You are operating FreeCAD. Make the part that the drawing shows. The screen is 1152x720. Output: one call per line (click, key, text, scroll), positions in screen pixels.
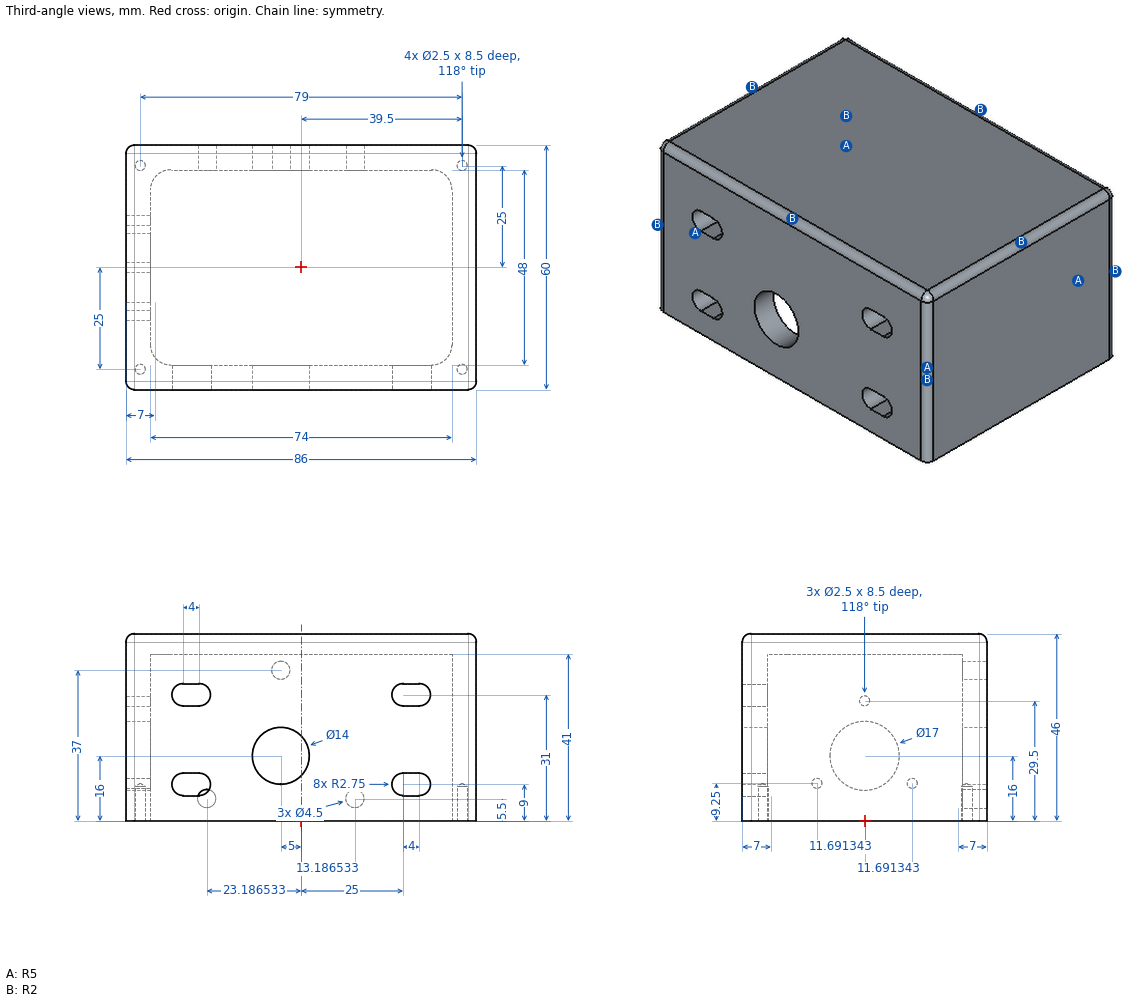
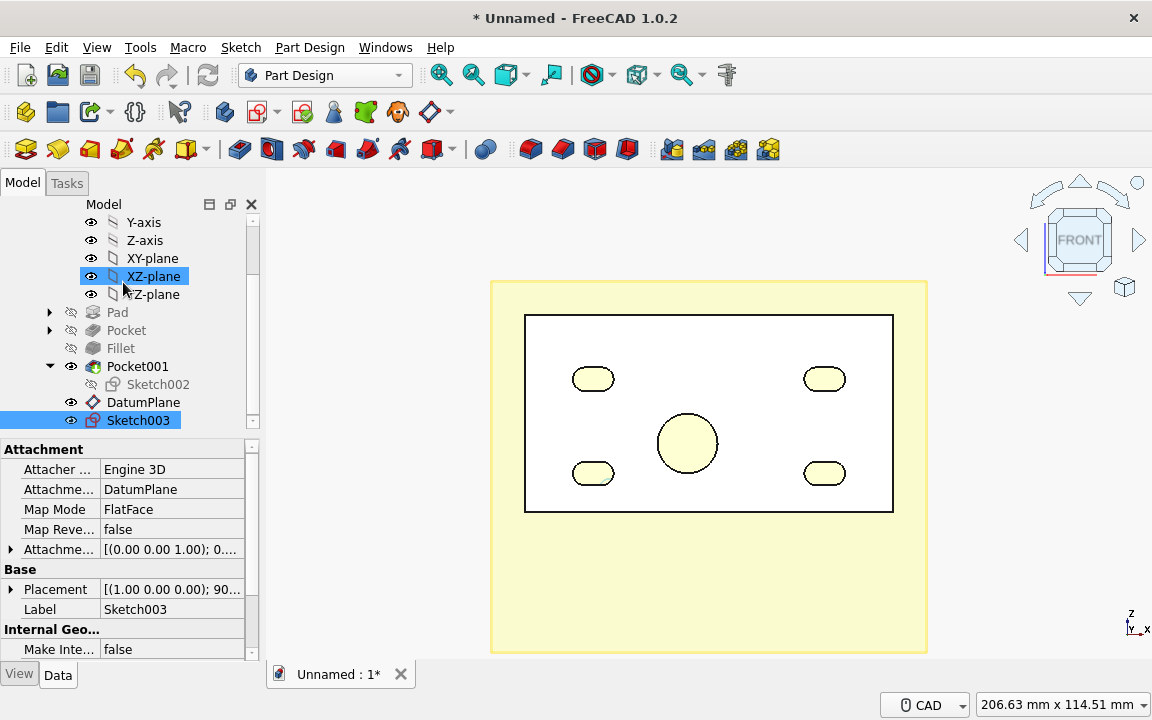
click(240, 150)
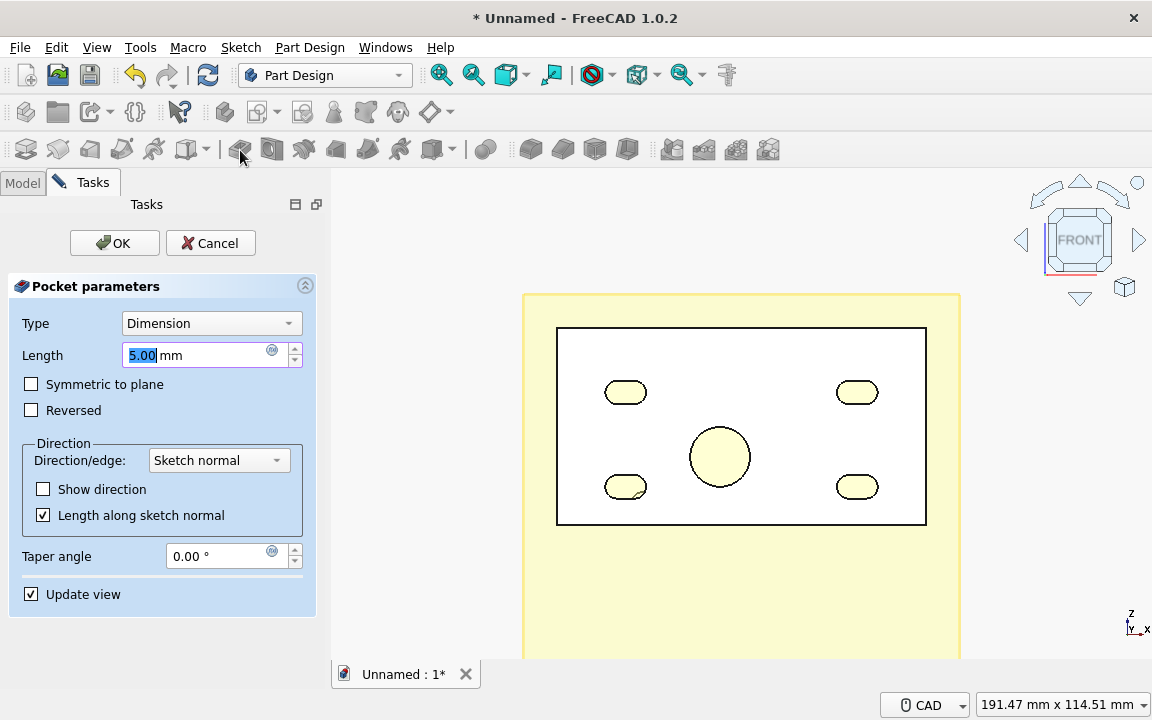
text(7)
key(Tab)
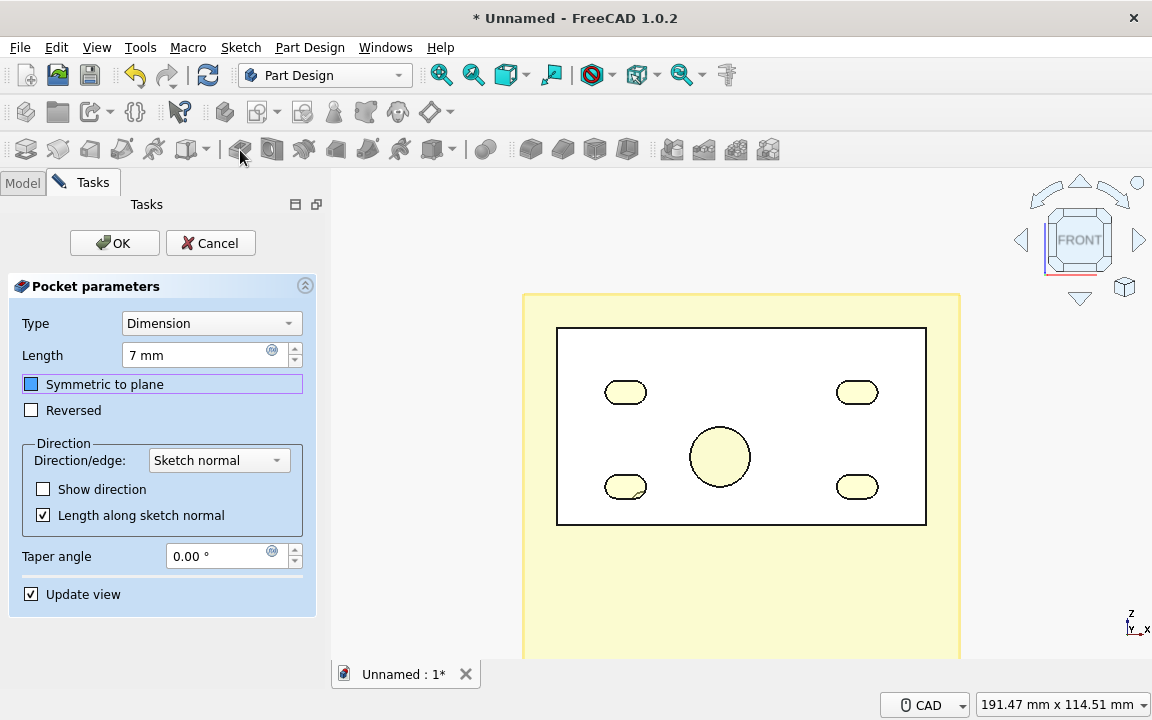
click(115, 243)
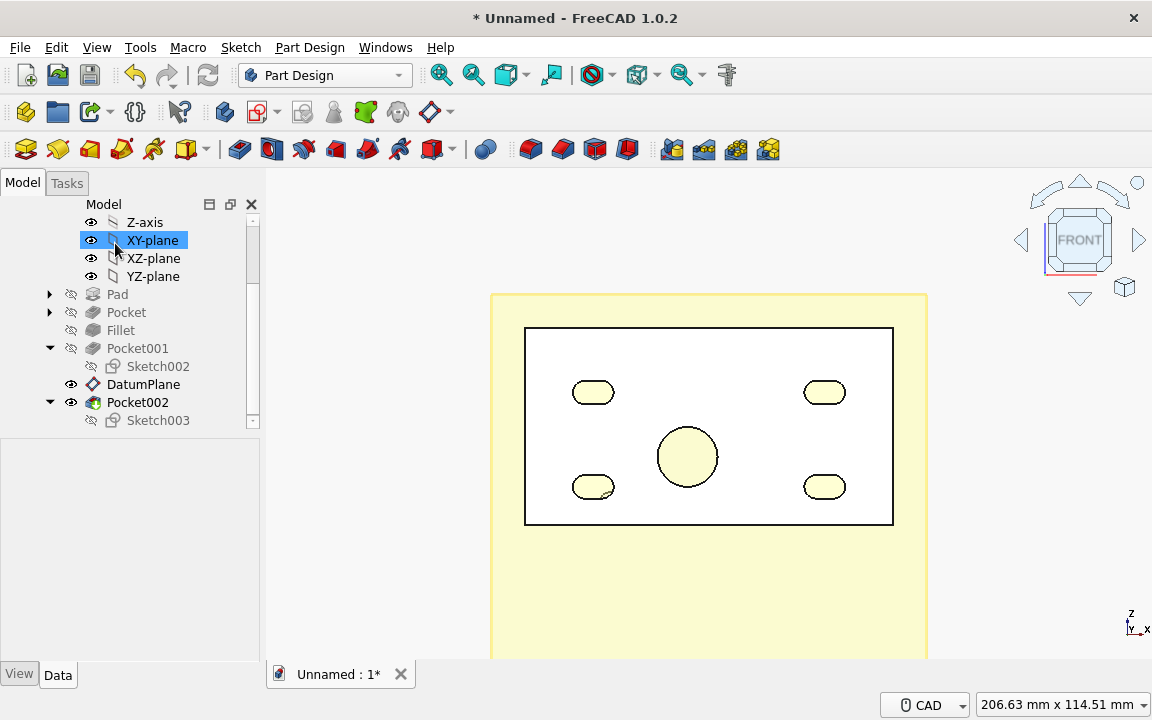
click(116, 384)
key(space)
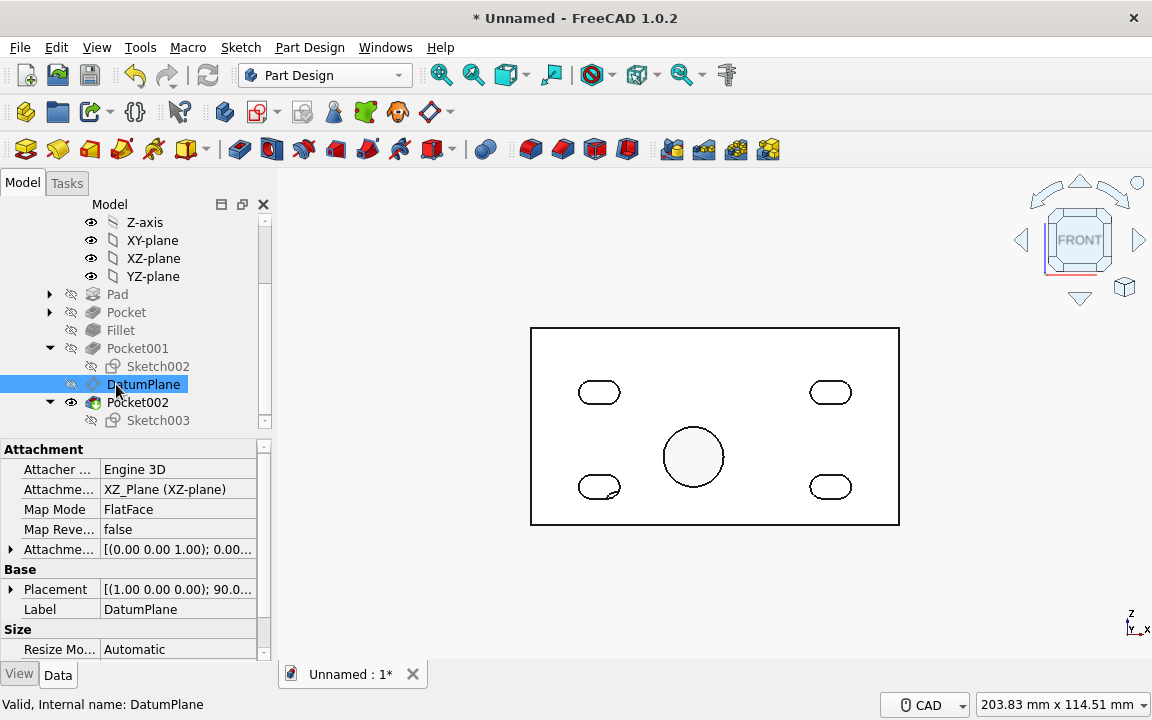
click(442, 76)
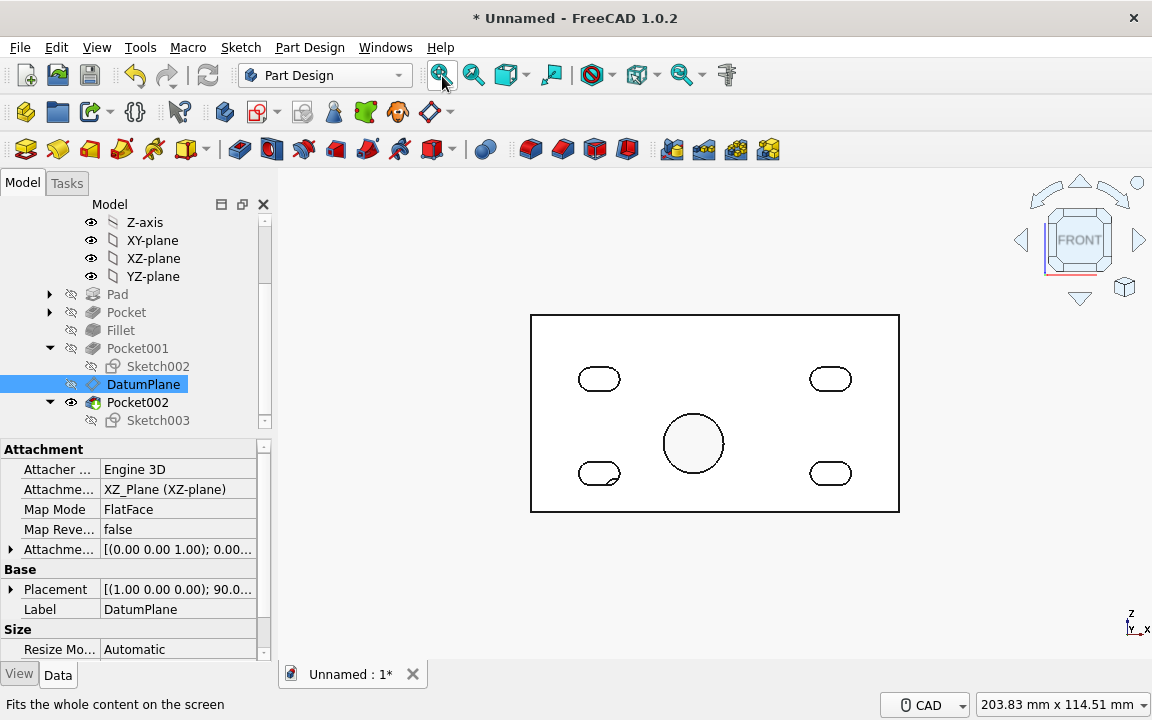
key(6)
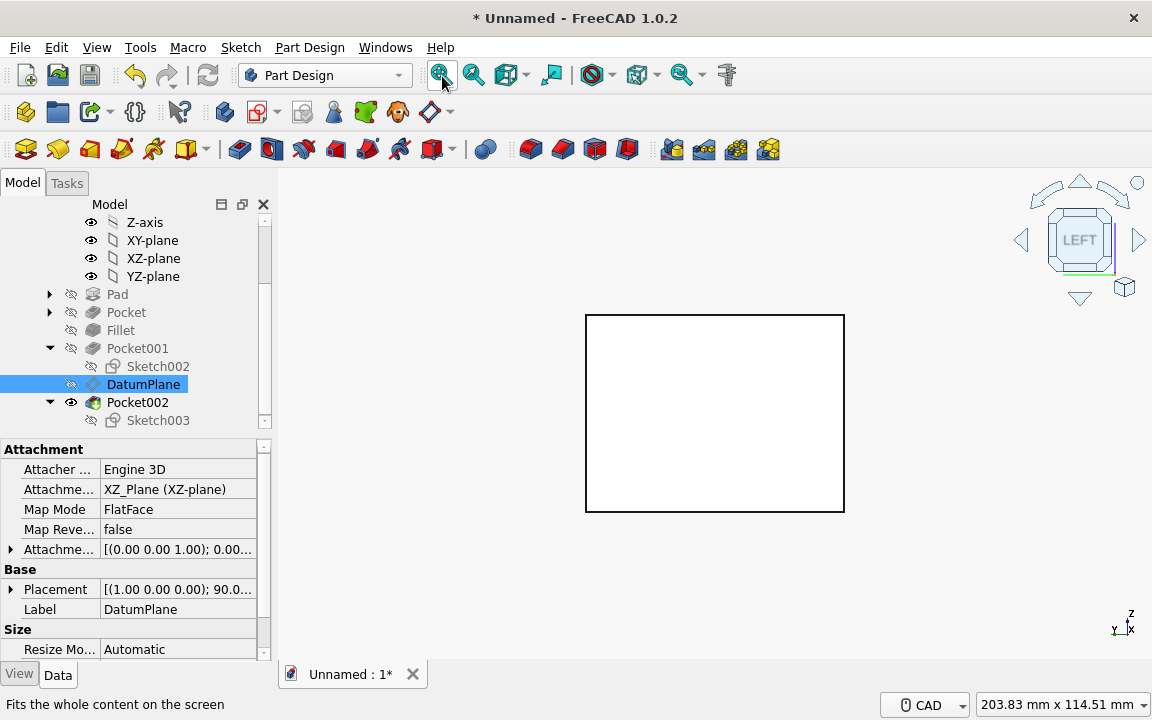
key(v)
key(f)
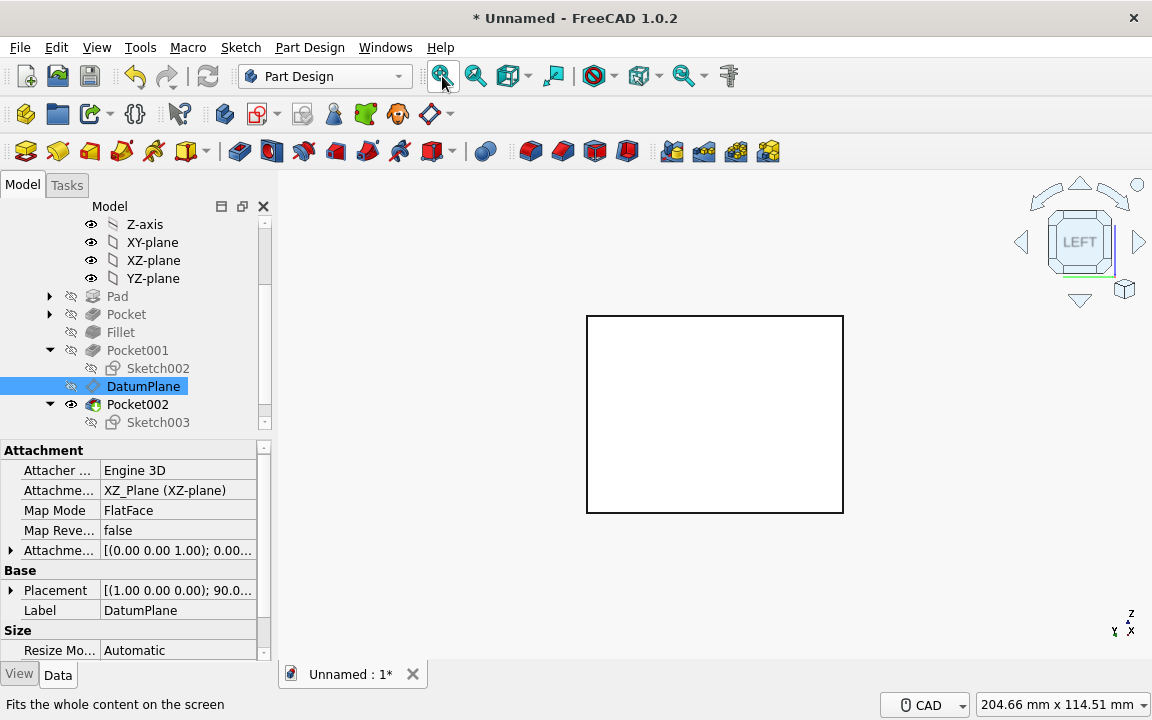
click(715, 413)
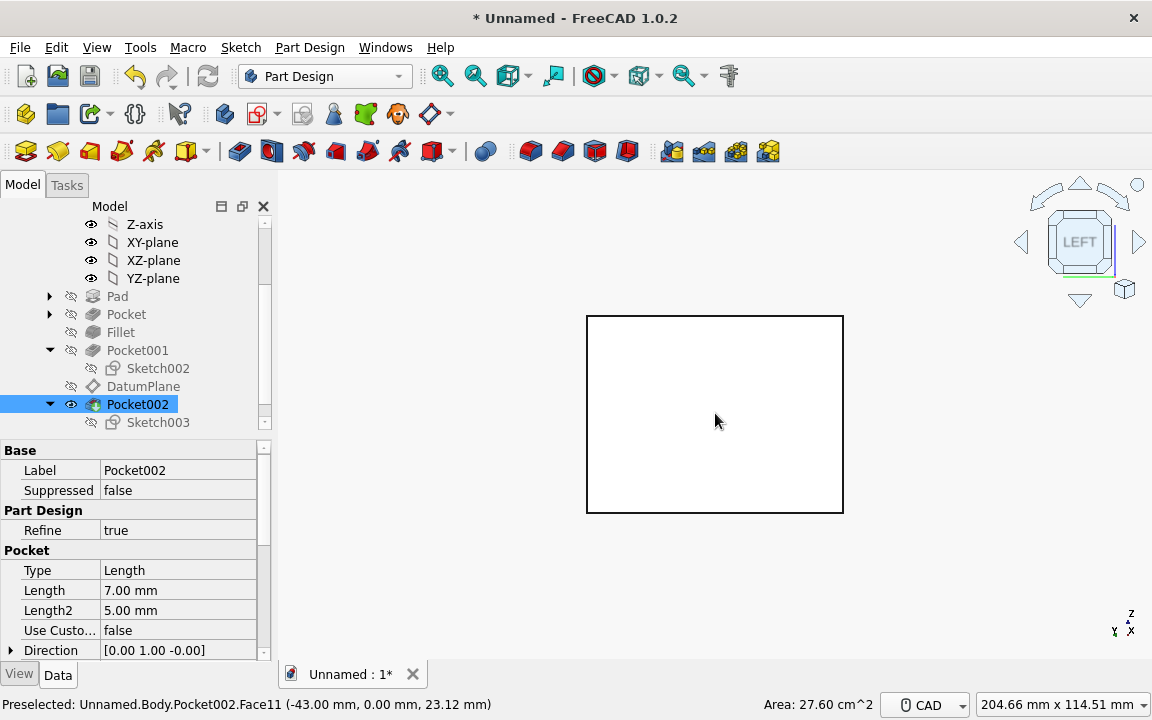
click(258, 114)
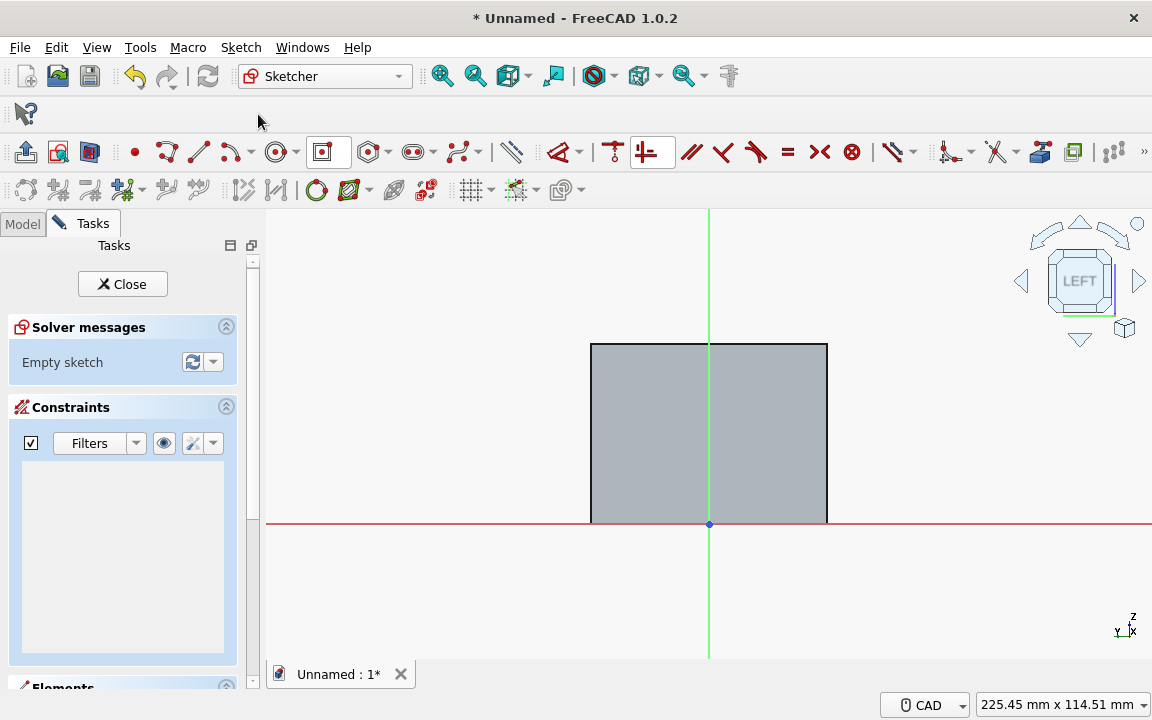
scroll(749, 501, up, 5)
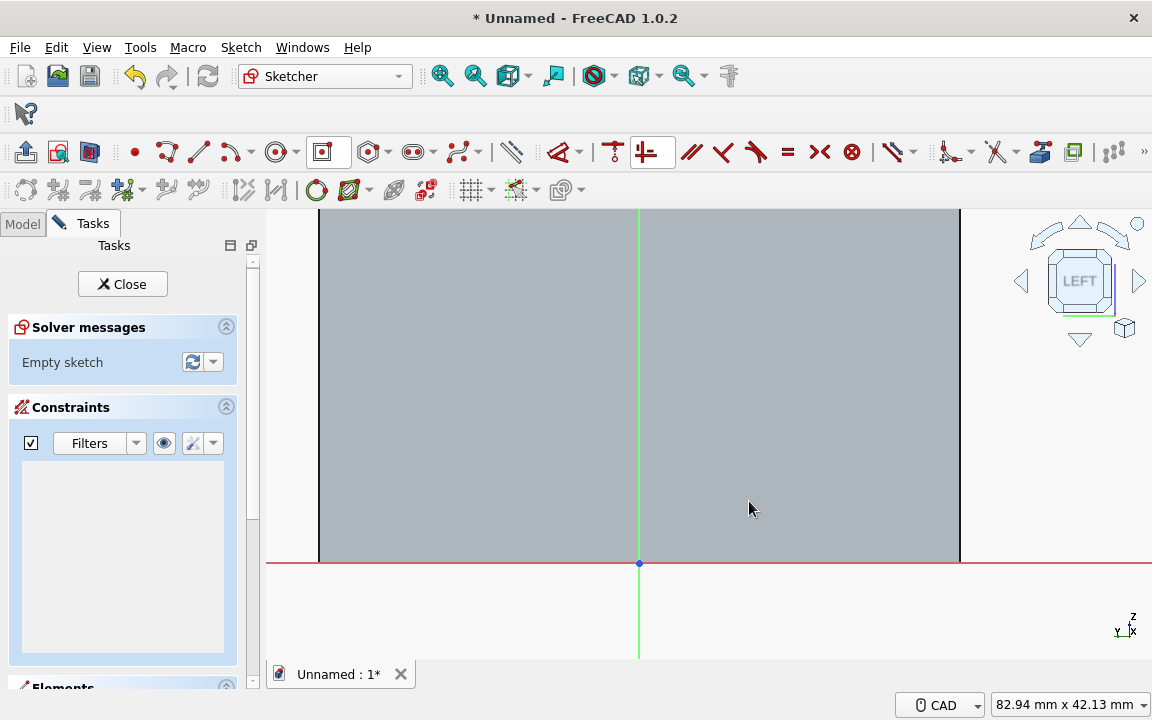
key(g)
key(c)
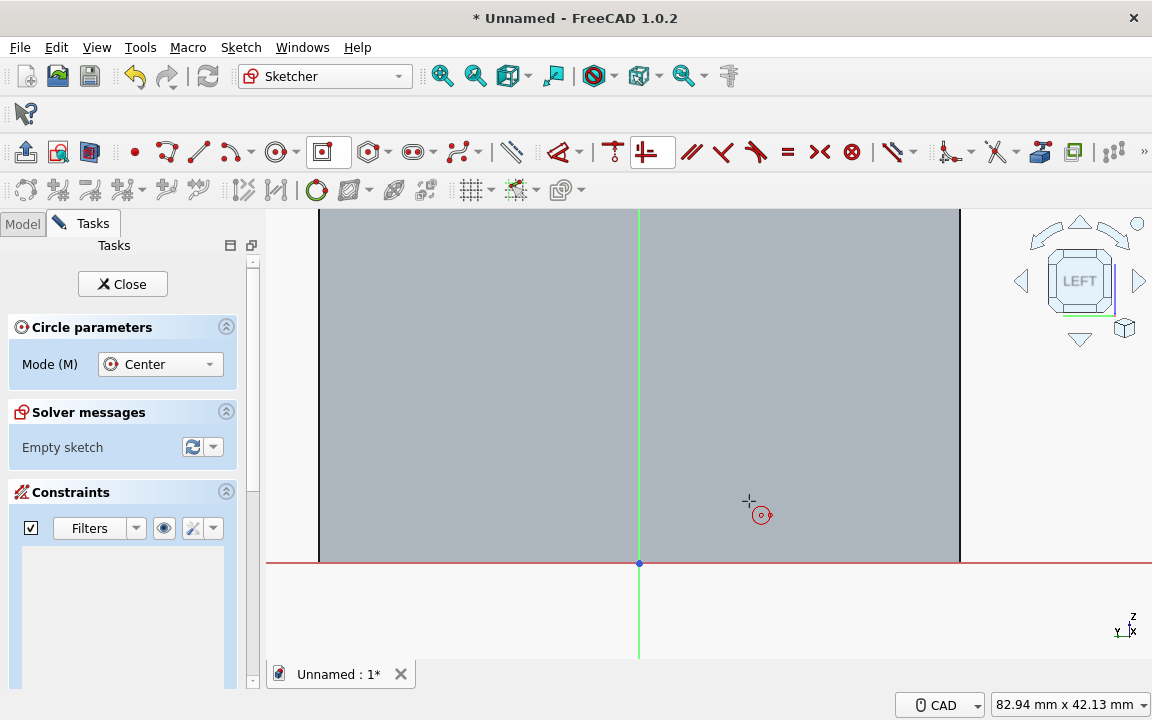
click(639, 393)
click(704, 328)
key(Escape)